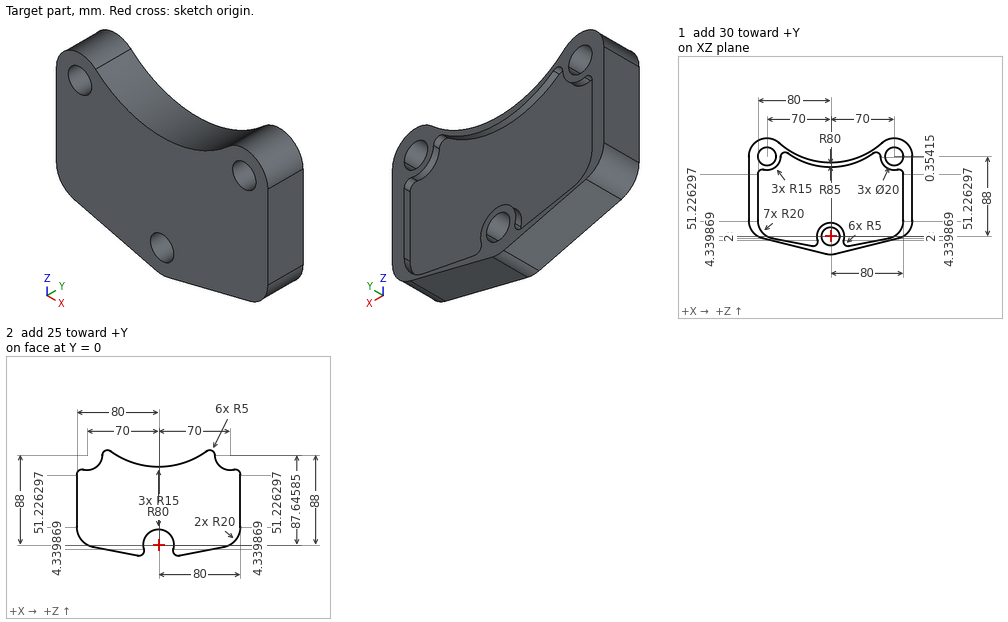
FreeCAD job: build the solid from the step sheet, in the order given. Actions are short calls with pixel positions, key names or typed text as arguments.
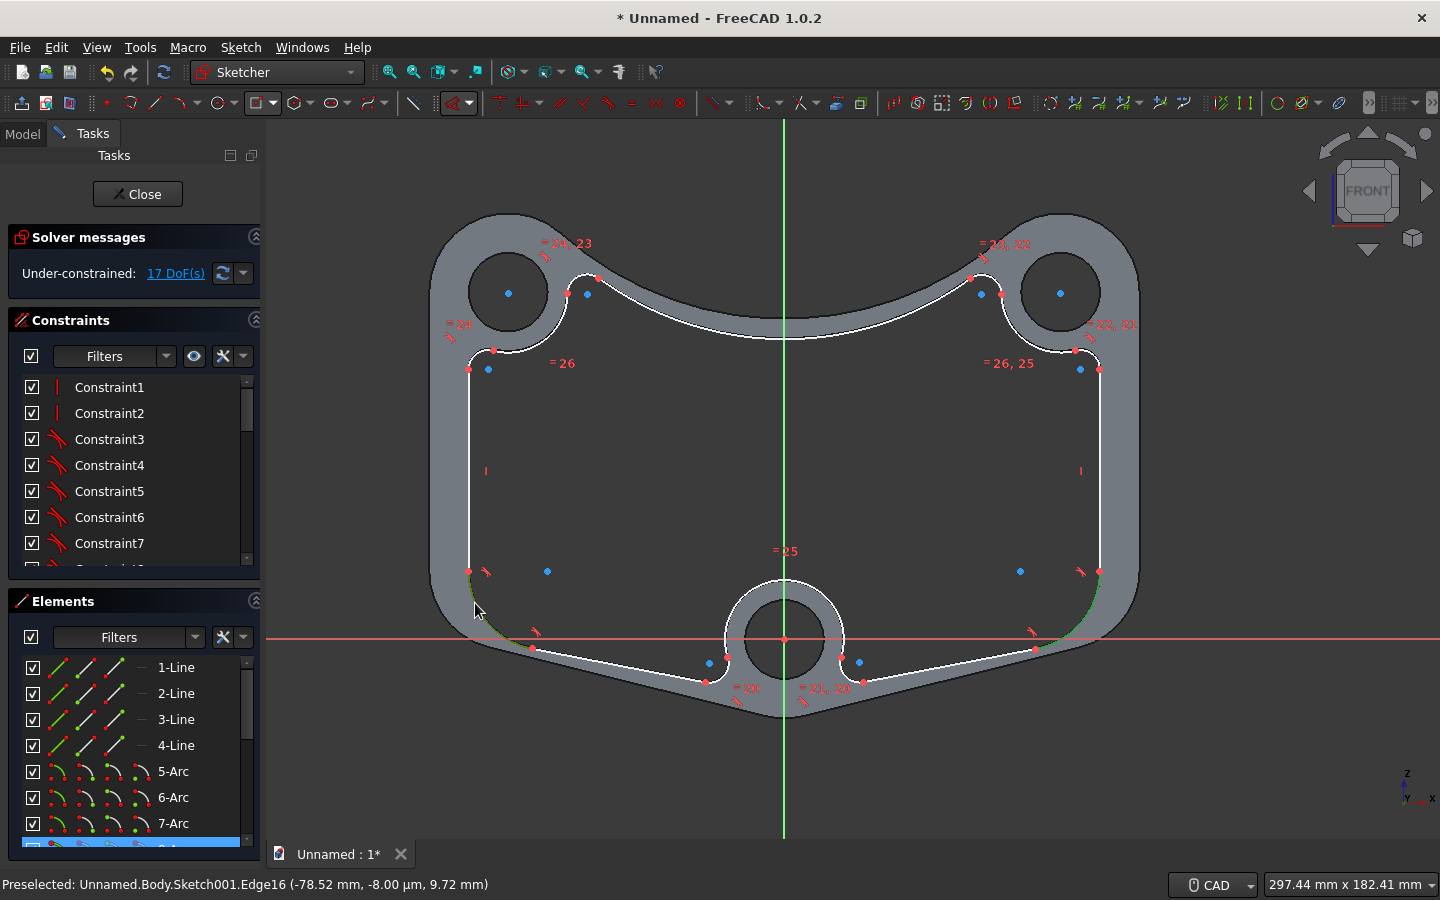
click(632, 104)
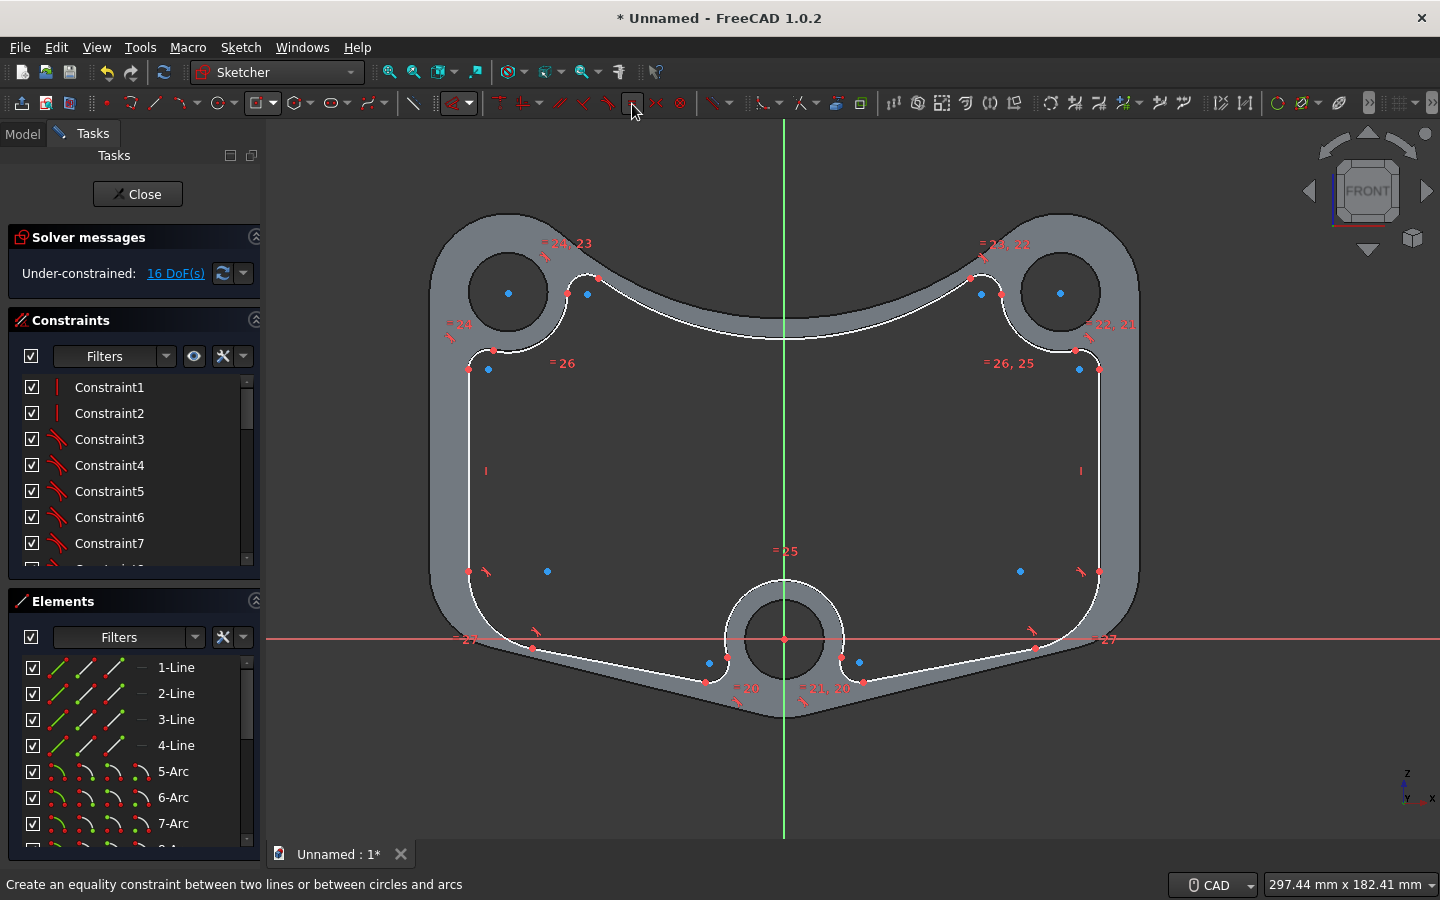
scroll(785, 735, down, 2)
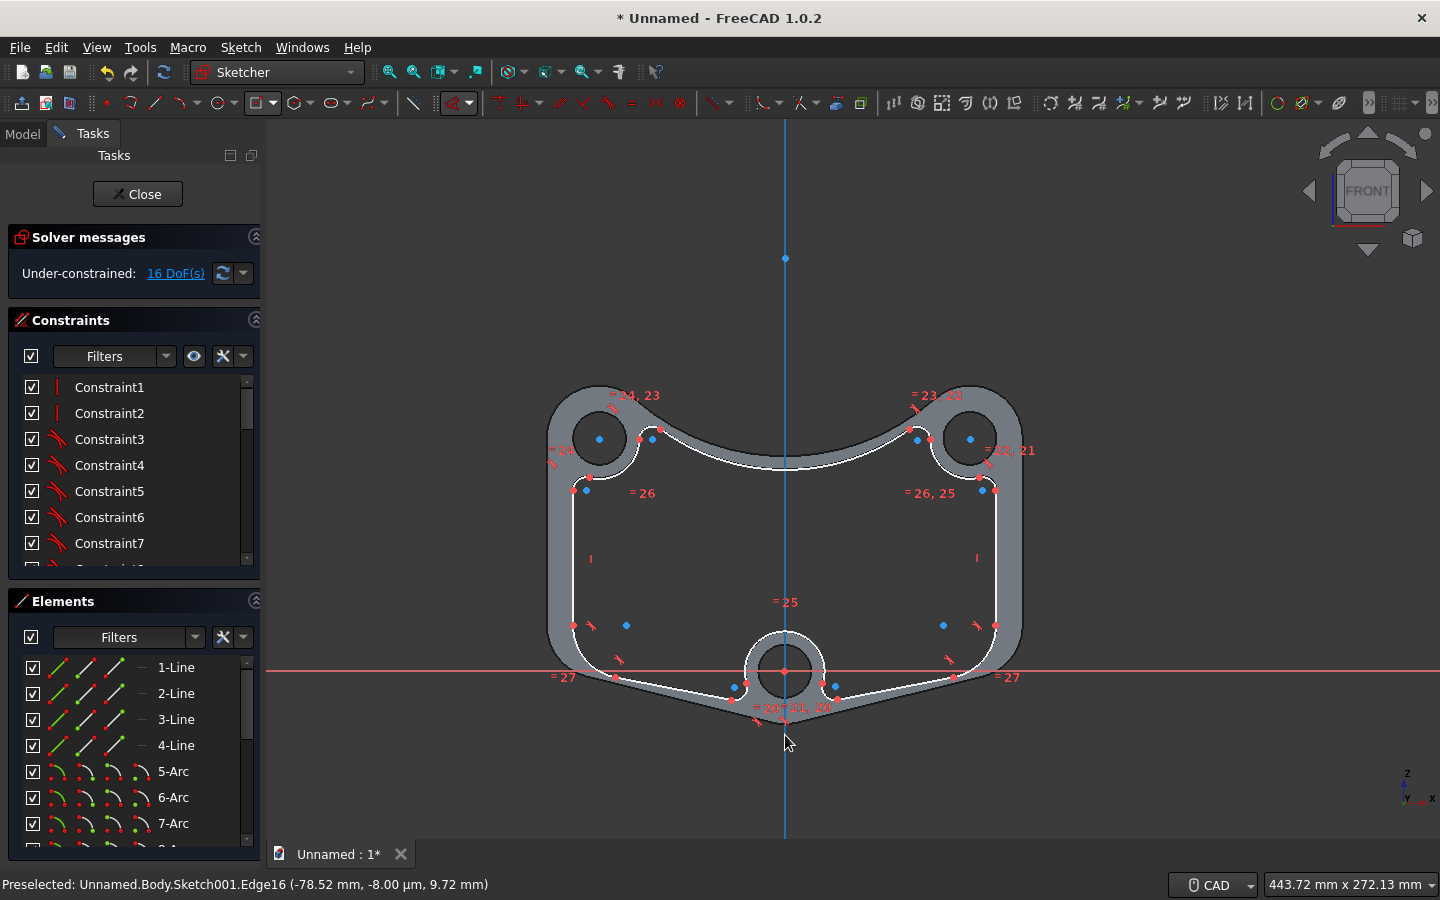
click(785, 259)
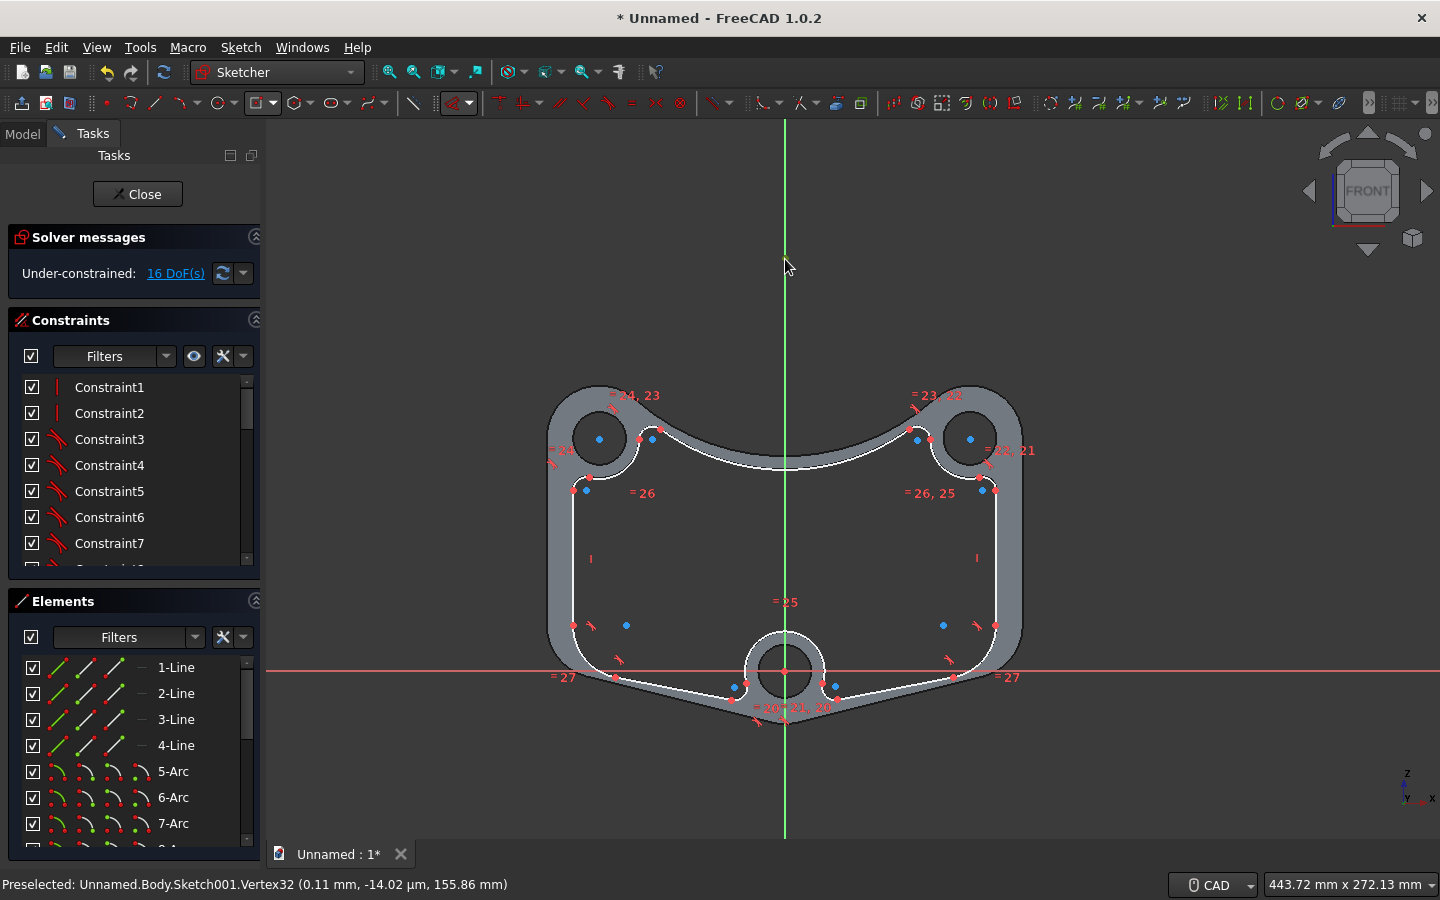
click(785, 764)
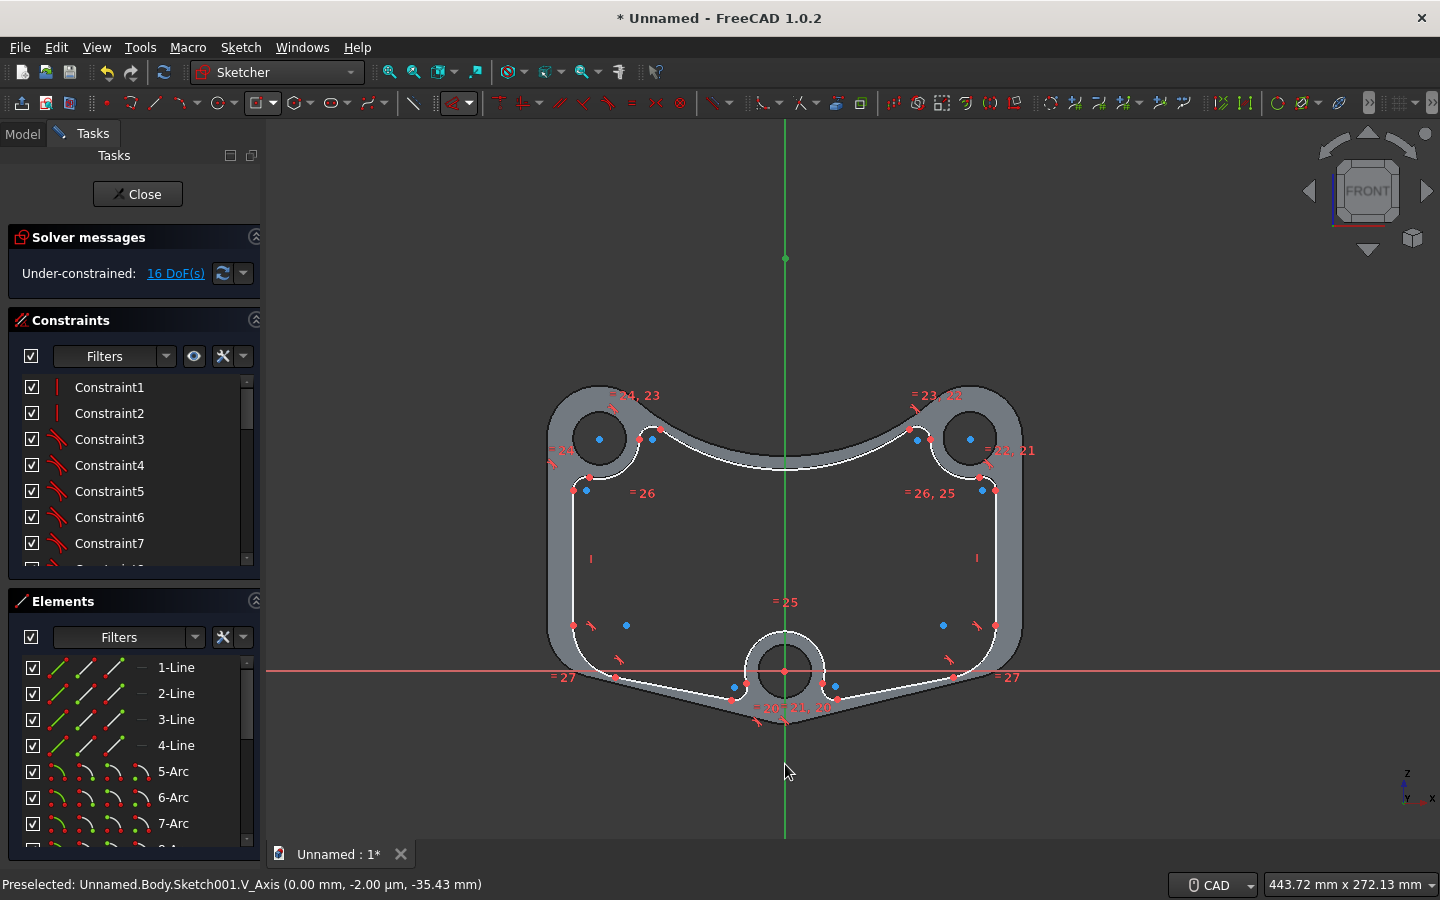
click(500, 104)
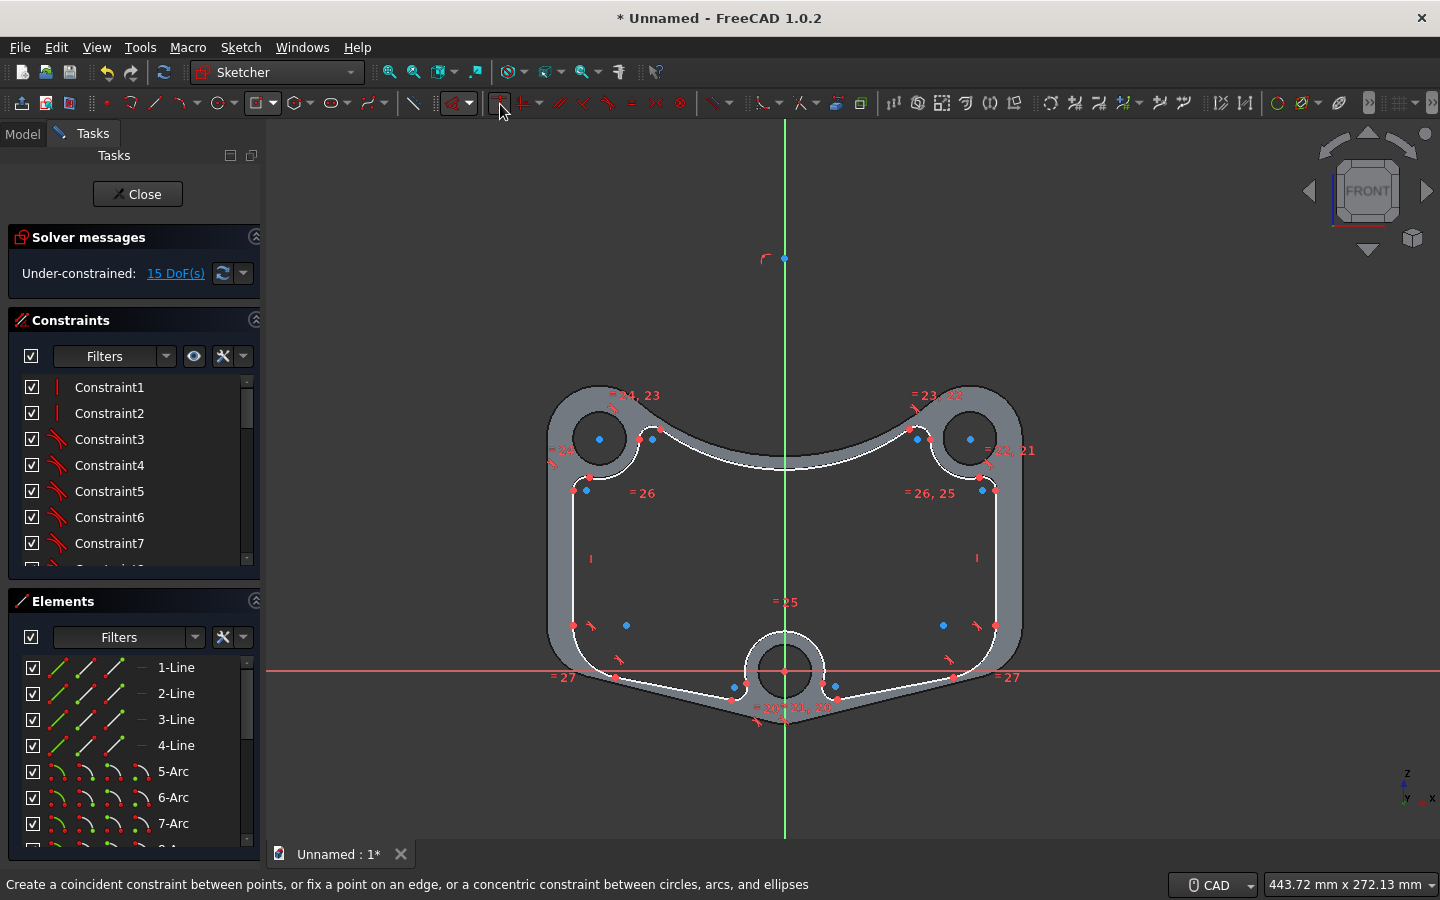
scroll(744, 696, up, 6)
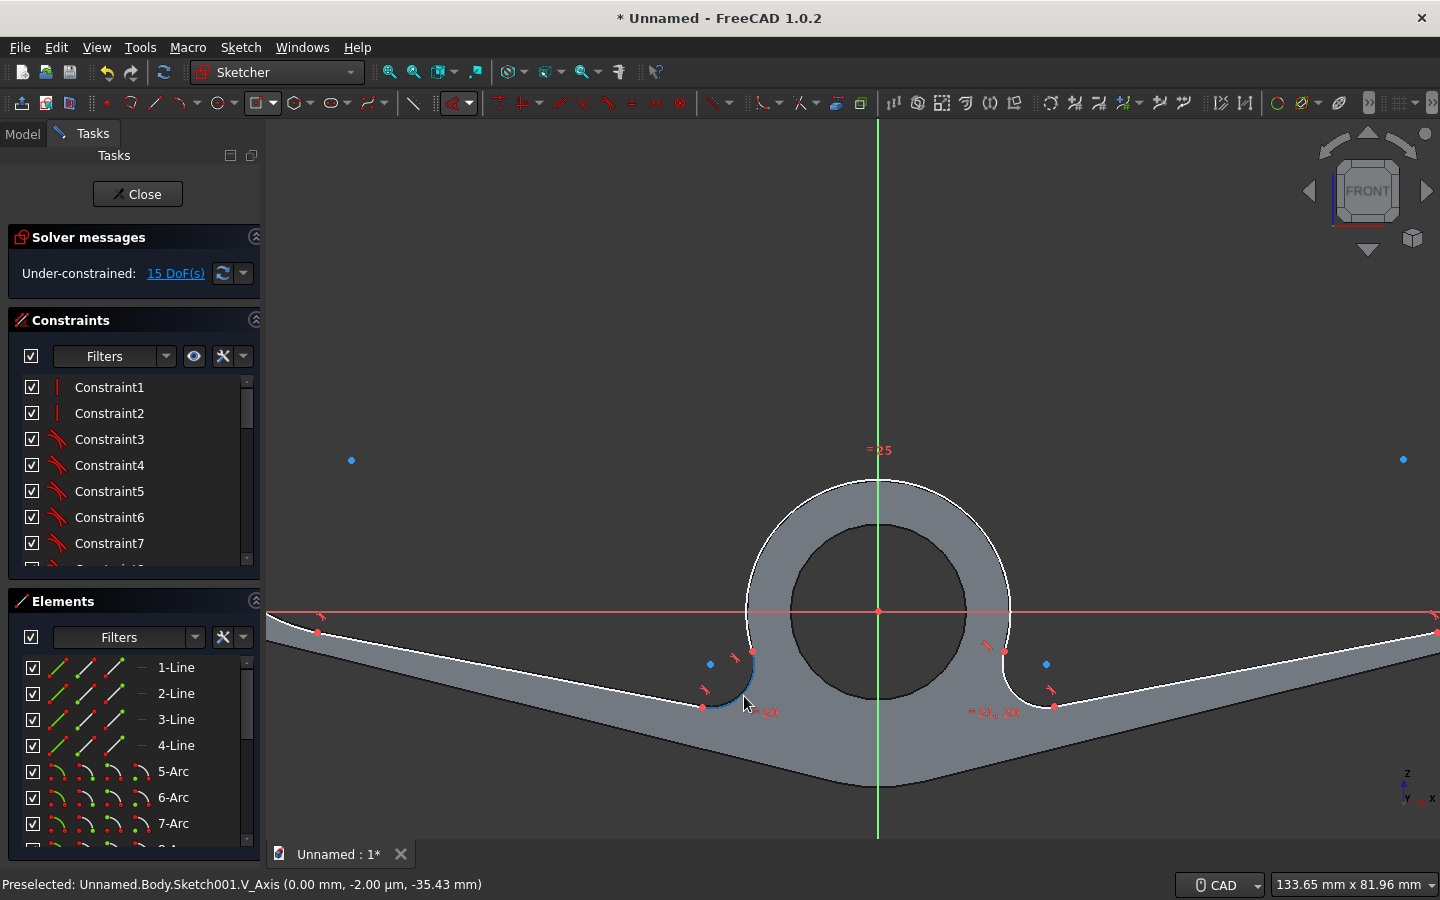
click(743, 694)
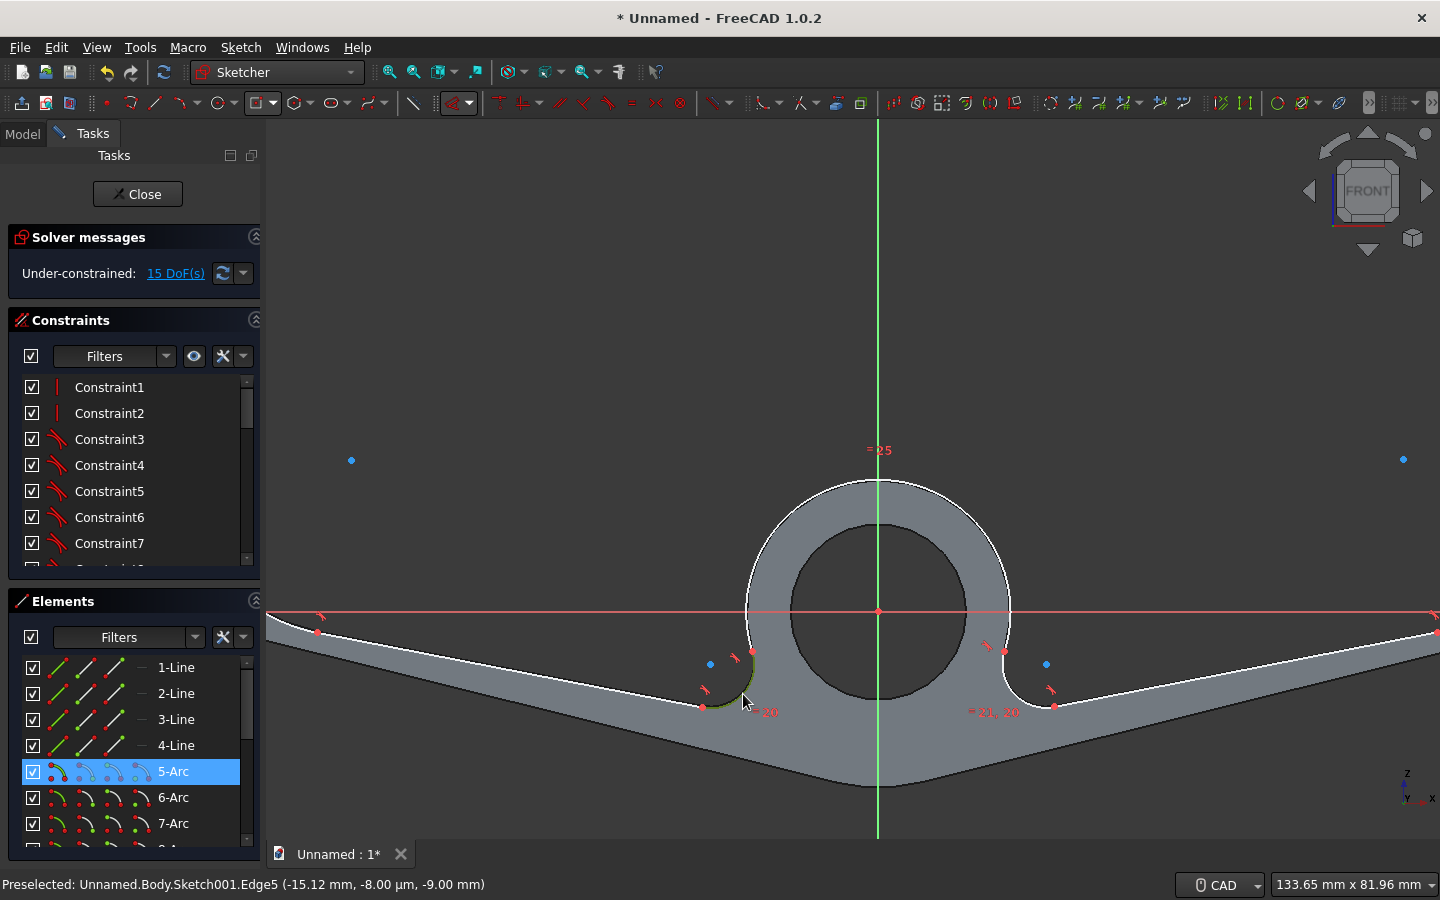
key(k)
key(r)